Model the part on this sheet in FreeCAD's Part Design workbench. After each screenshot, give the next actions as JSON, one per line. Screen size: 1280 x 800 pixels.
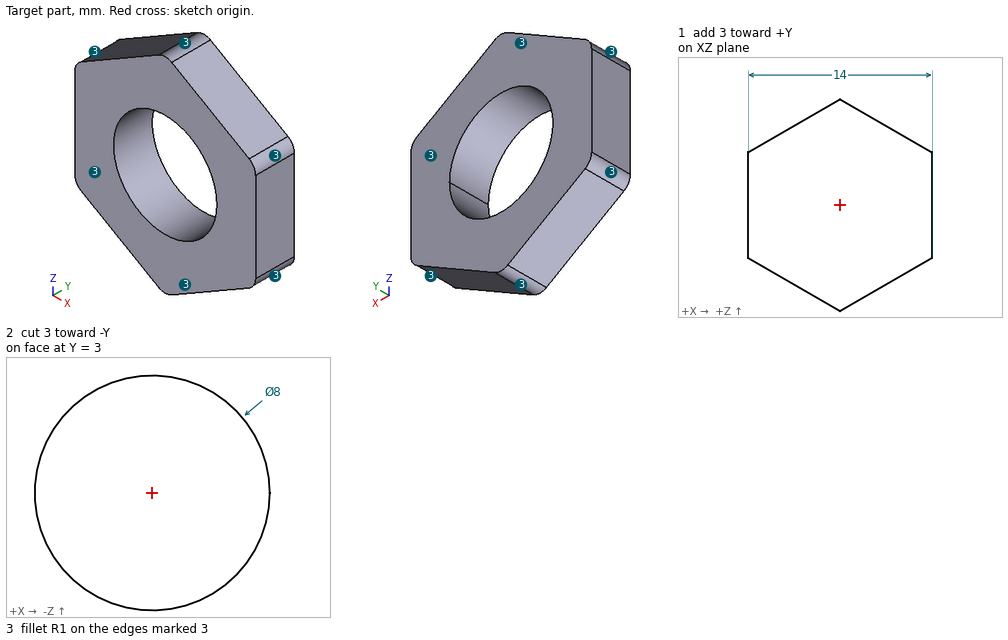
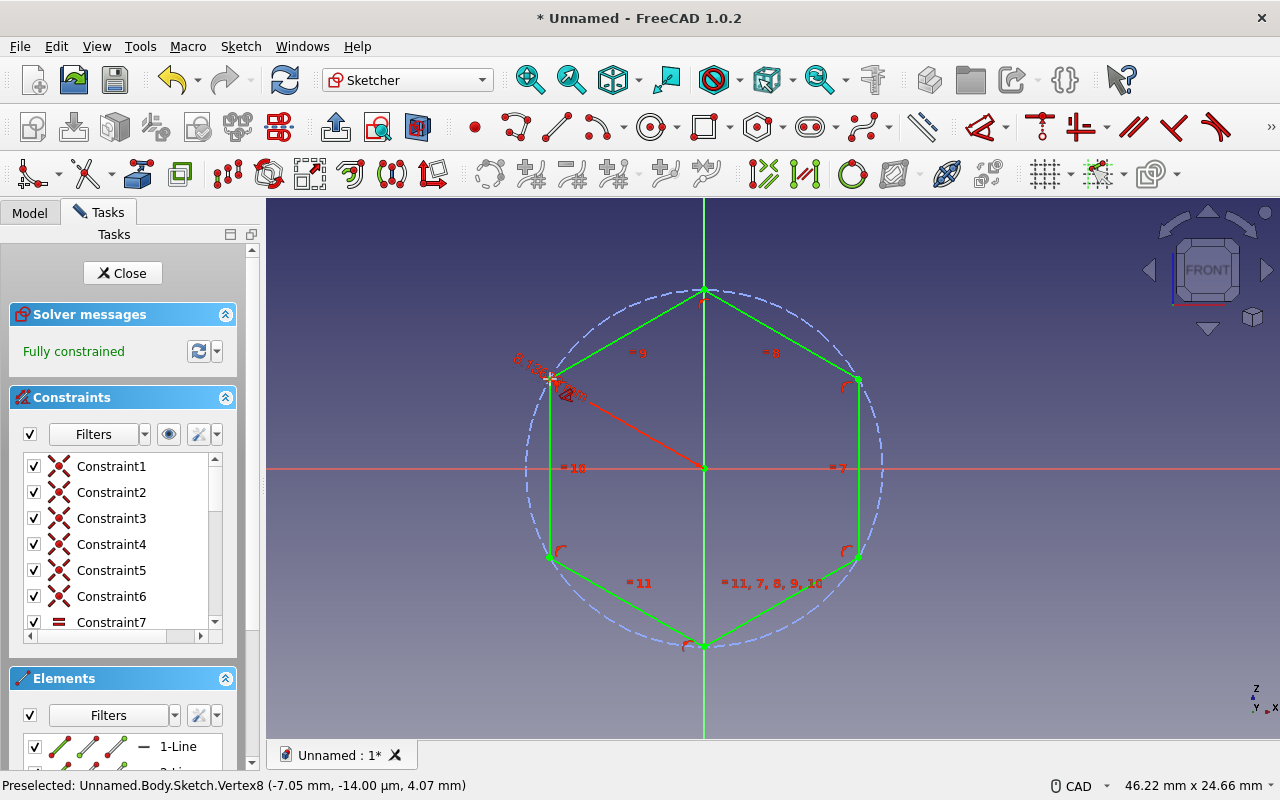
{"action": "left_click", "coordinate": [859, 558]}
{"action": "left_click", "coordinate": [596, 640]}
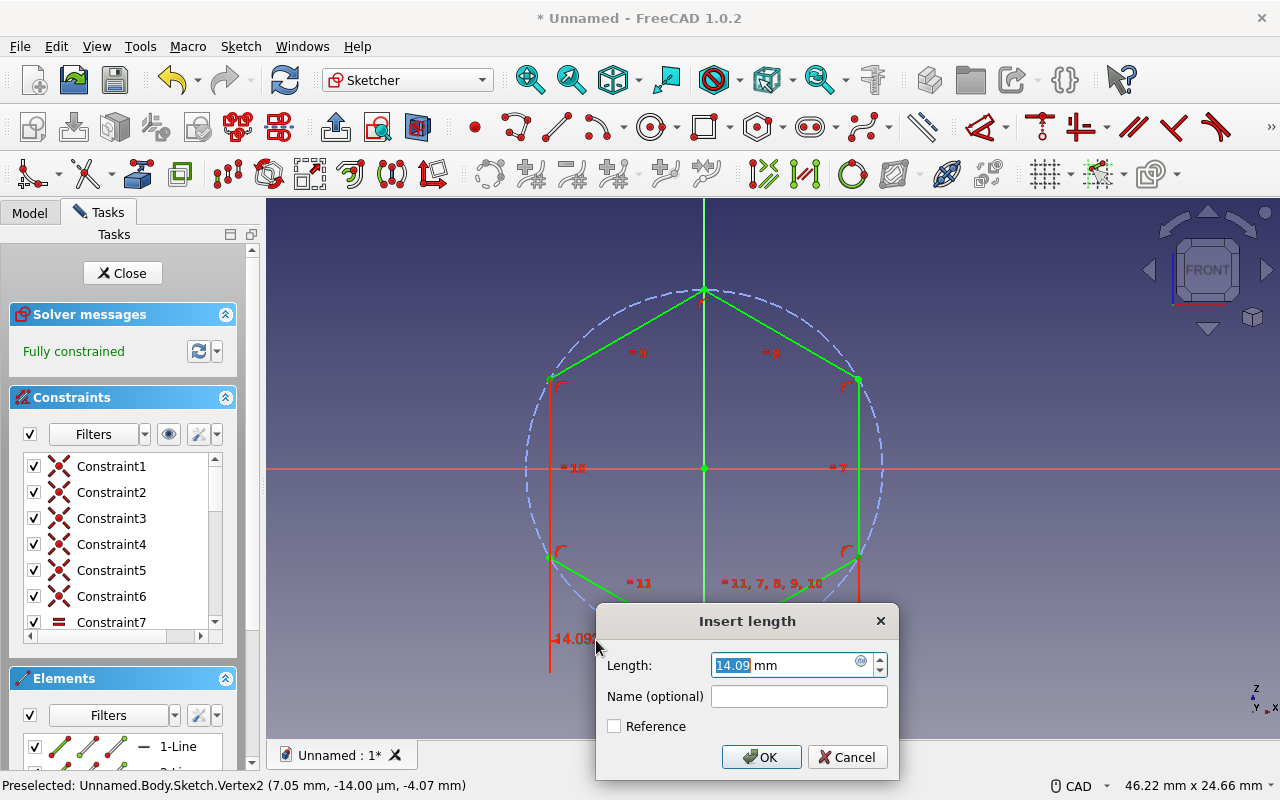
{"action": "type", "text": "14"}
{"action": "key", "text": "Return"}
{"action": "key", "text": "Escape"}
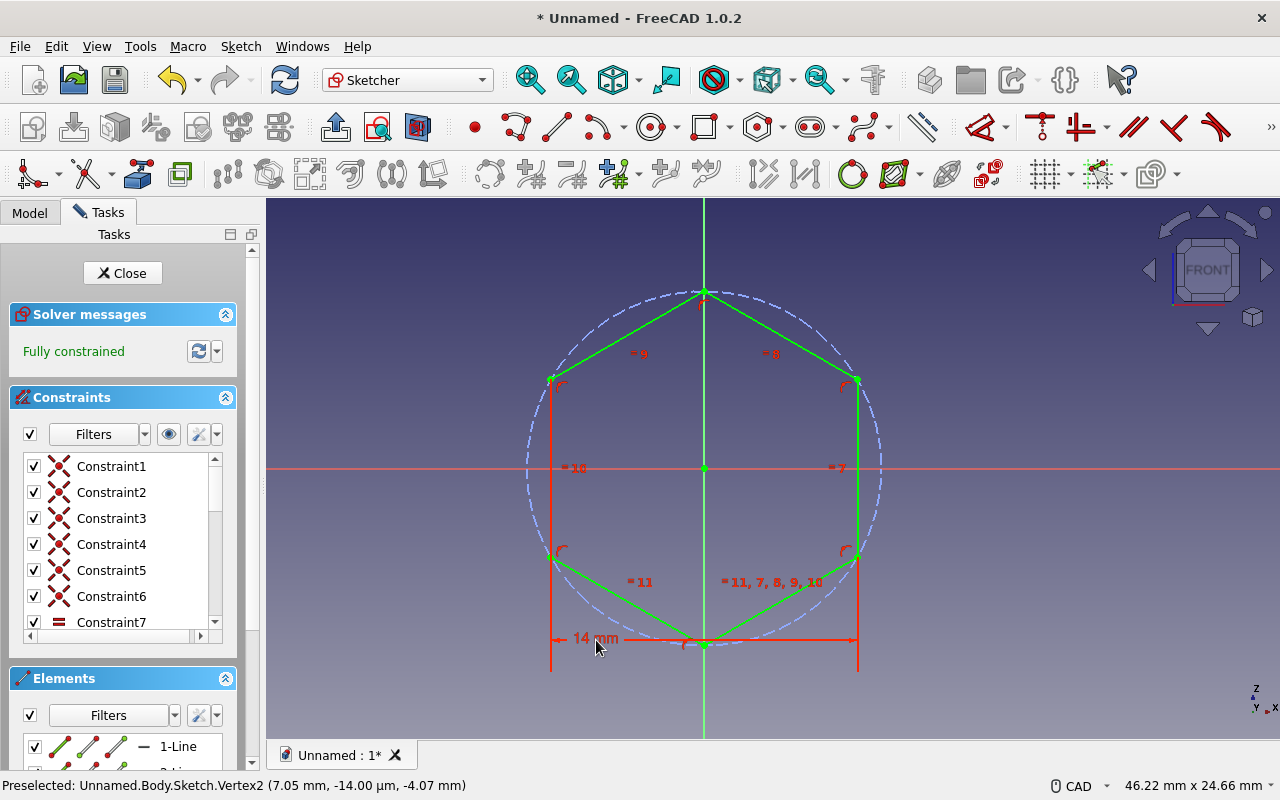
{"action": "left_click", "coordinate": [123, 273]}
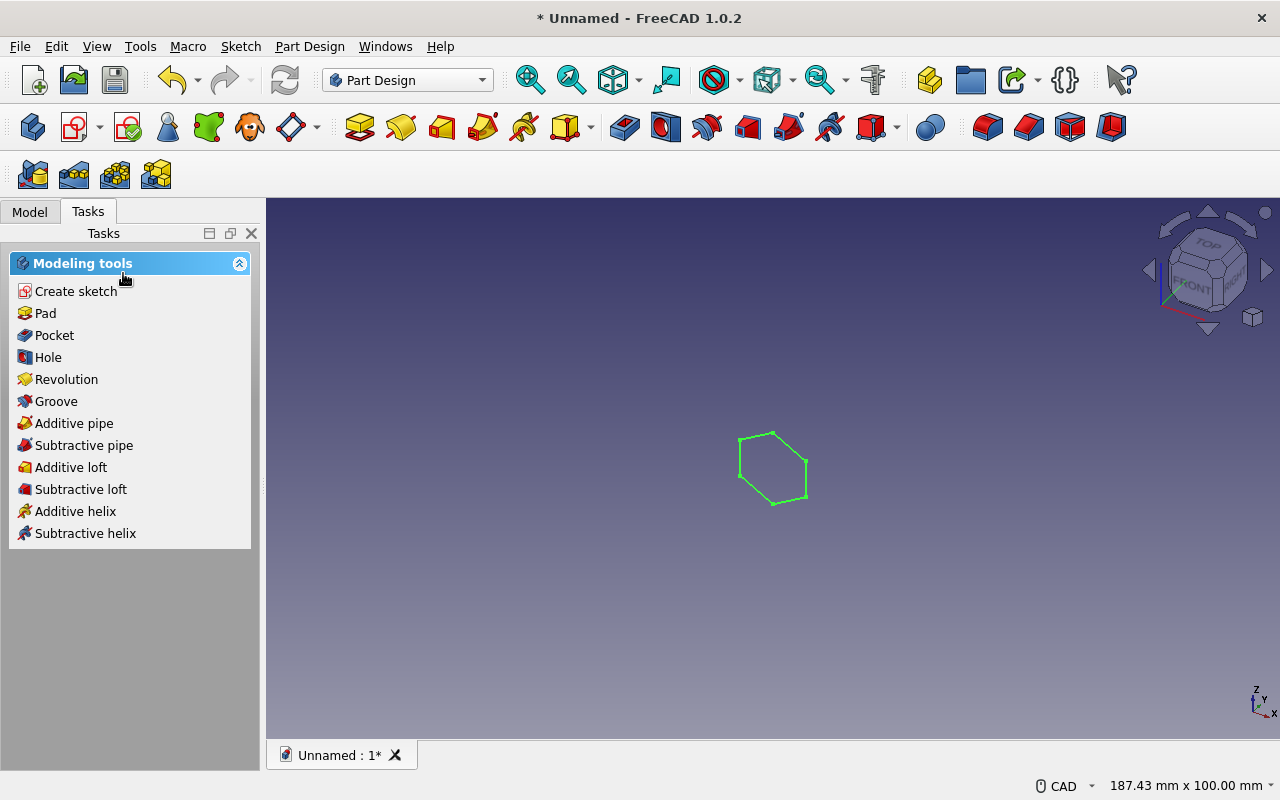
{"action": "left_click", "coordinate": [360, 128]}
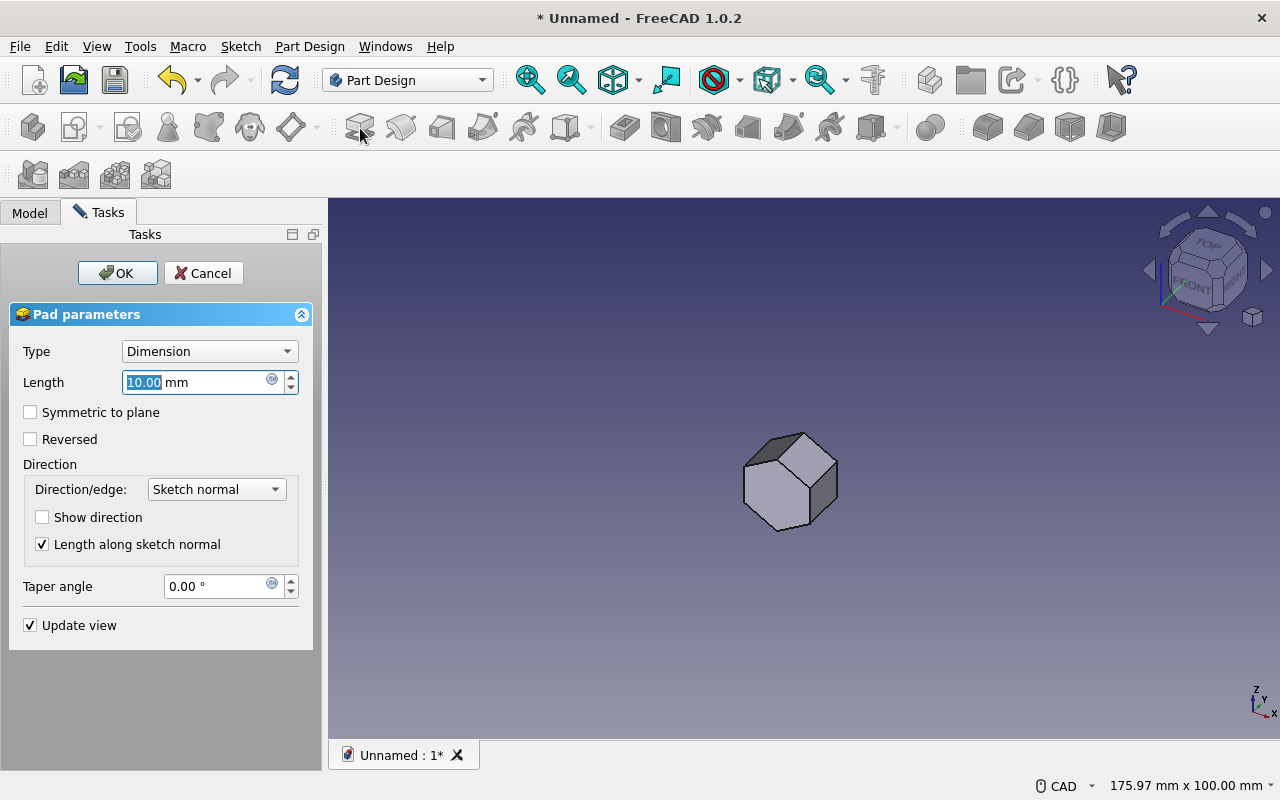
{"action": "type", "text": "3"}
{"action": "key", "text": "Tab"}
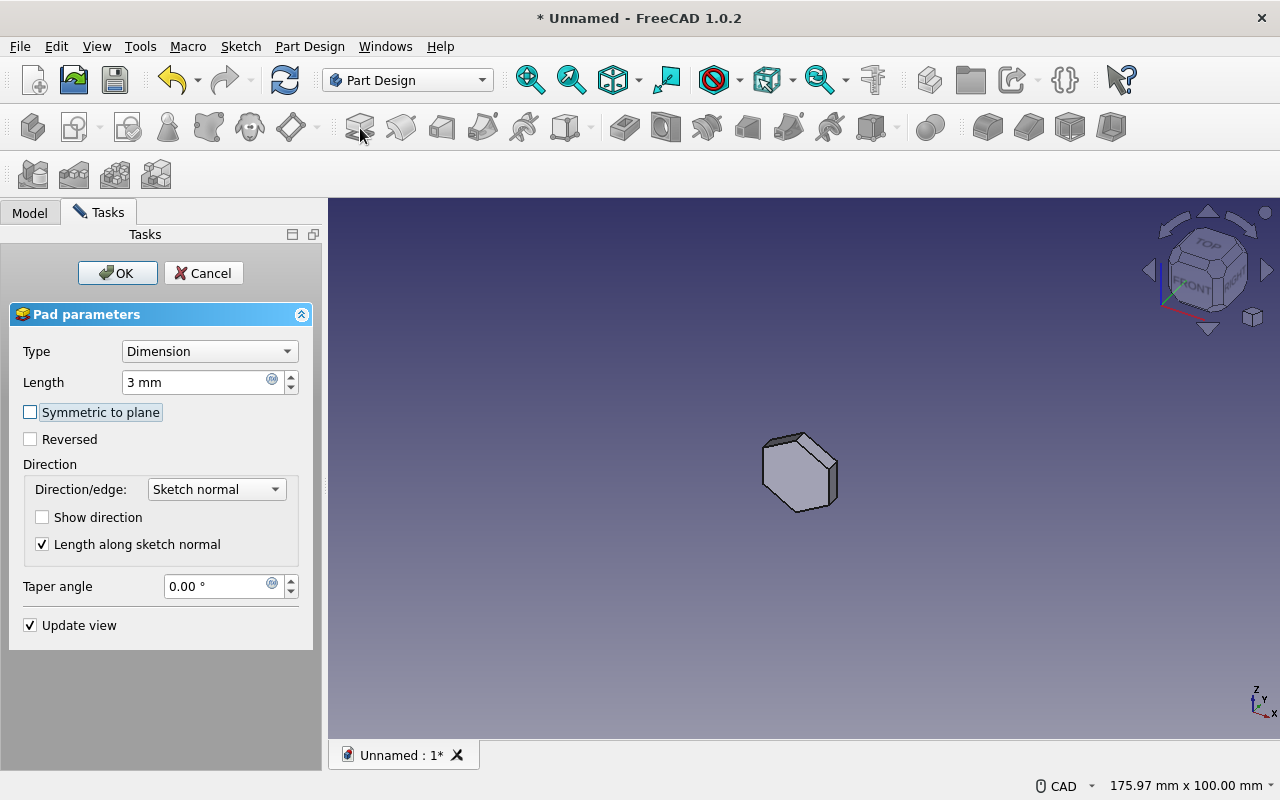
{"action": "left_click", "coordinate": [31, 439]}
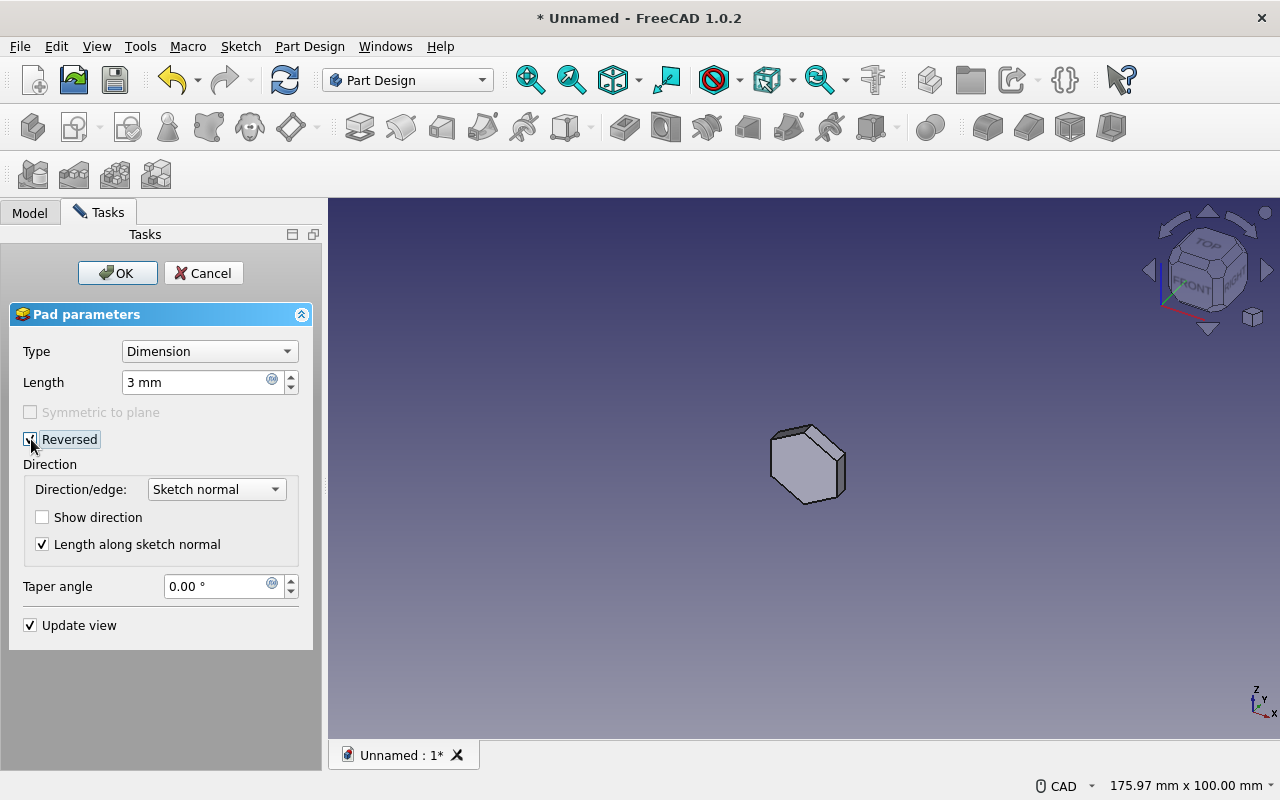
{"action": "left_click", "coordinate": [118, 273]}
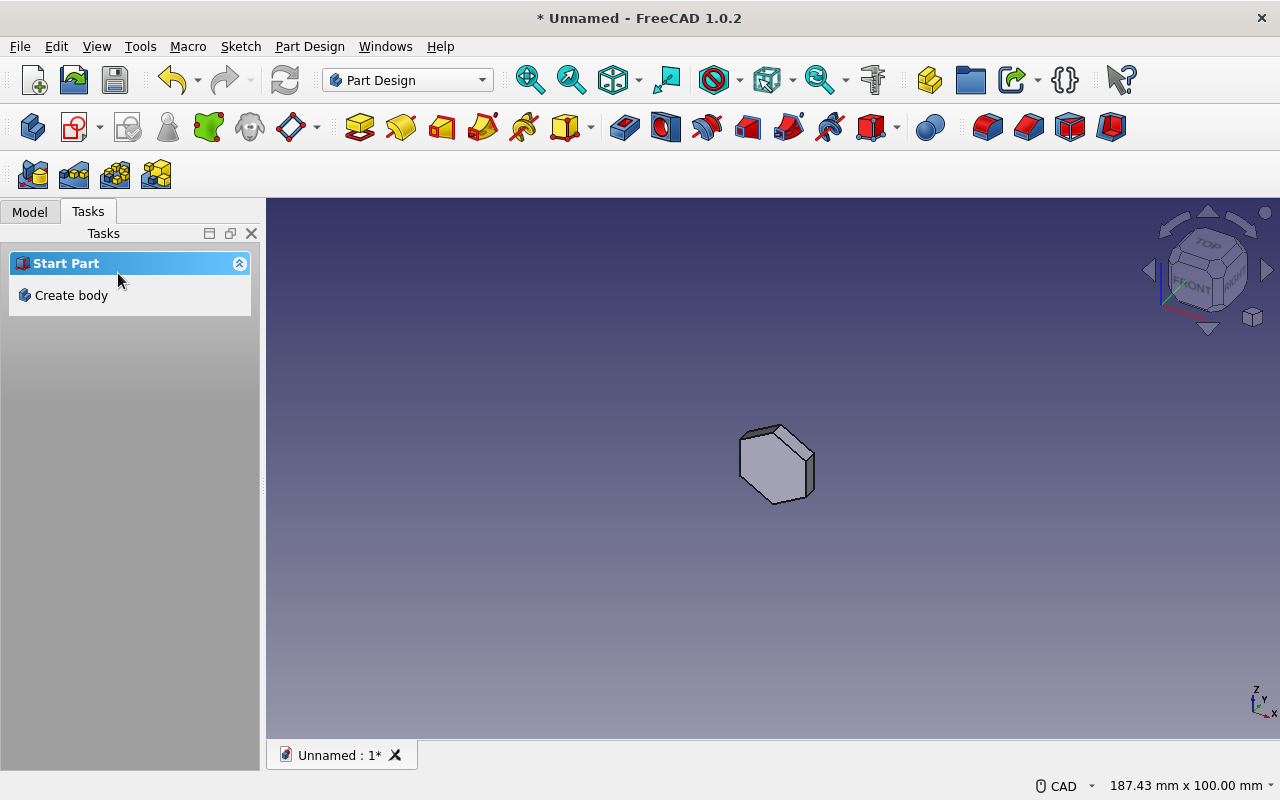
{"action": "key", "text": "v f"}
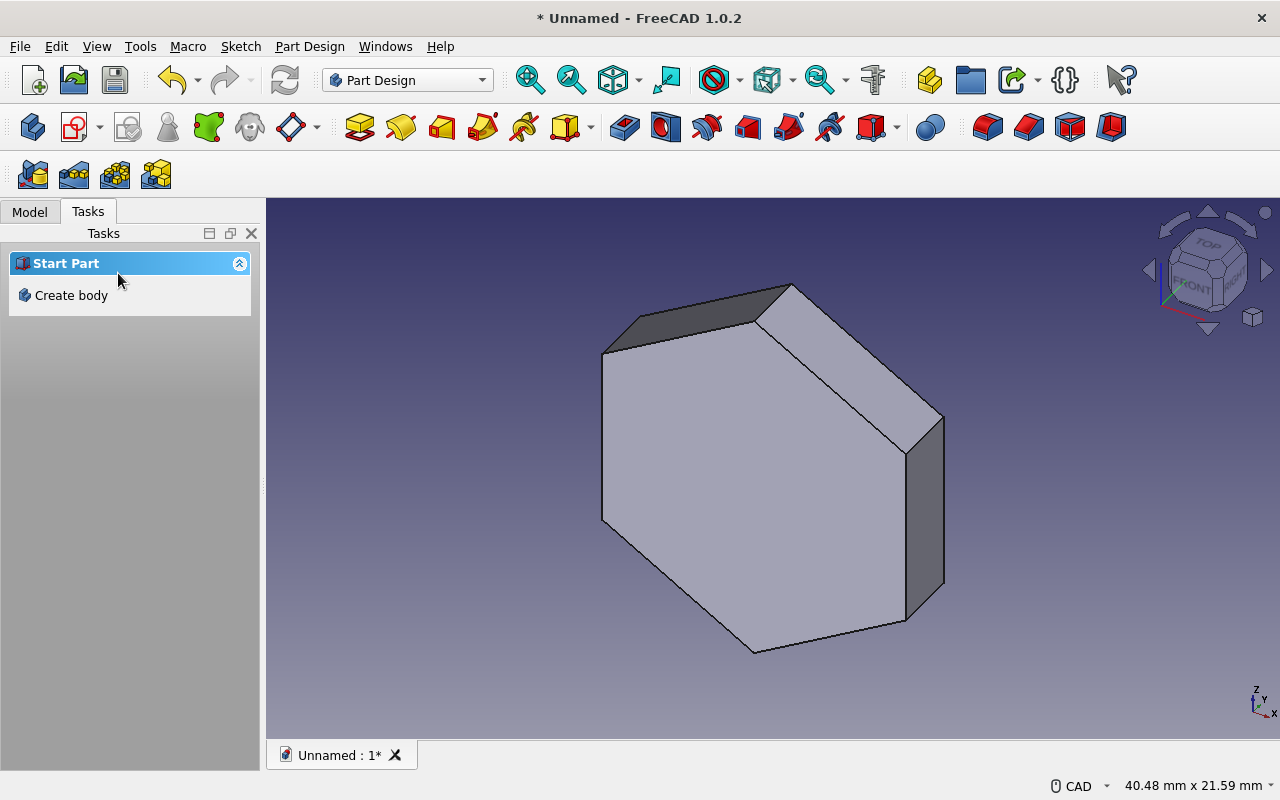
{"action": "key", "text": "4"}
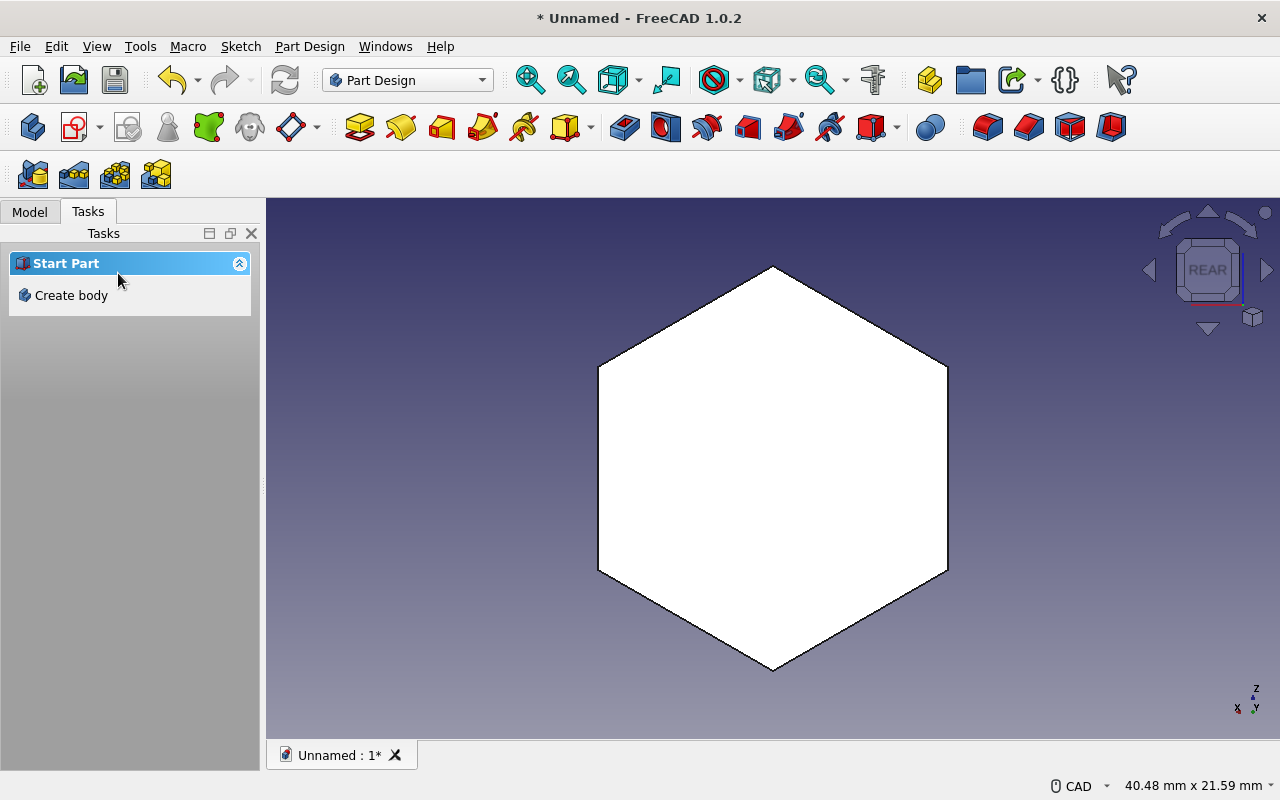
{"action": "left_click", "coordinate": [773, 468]}